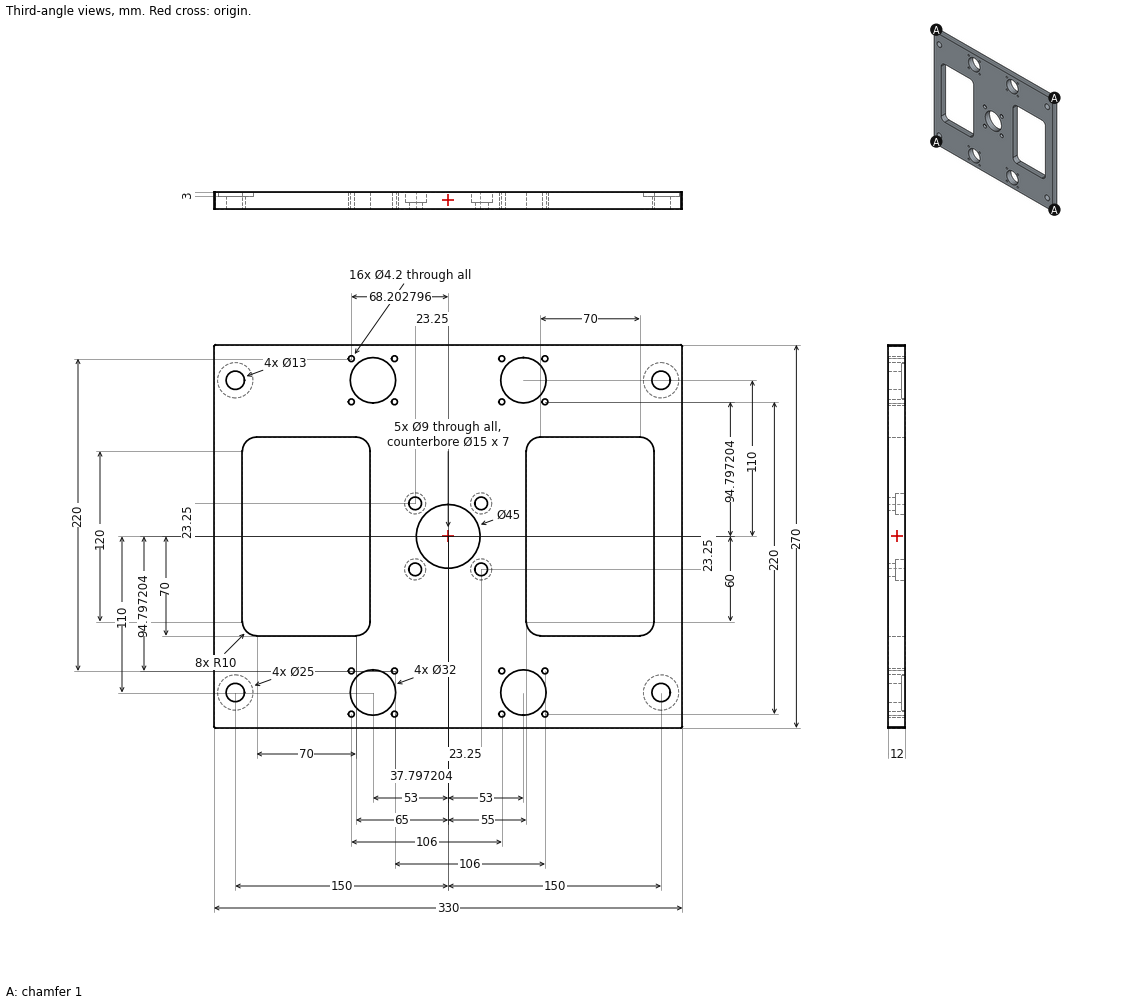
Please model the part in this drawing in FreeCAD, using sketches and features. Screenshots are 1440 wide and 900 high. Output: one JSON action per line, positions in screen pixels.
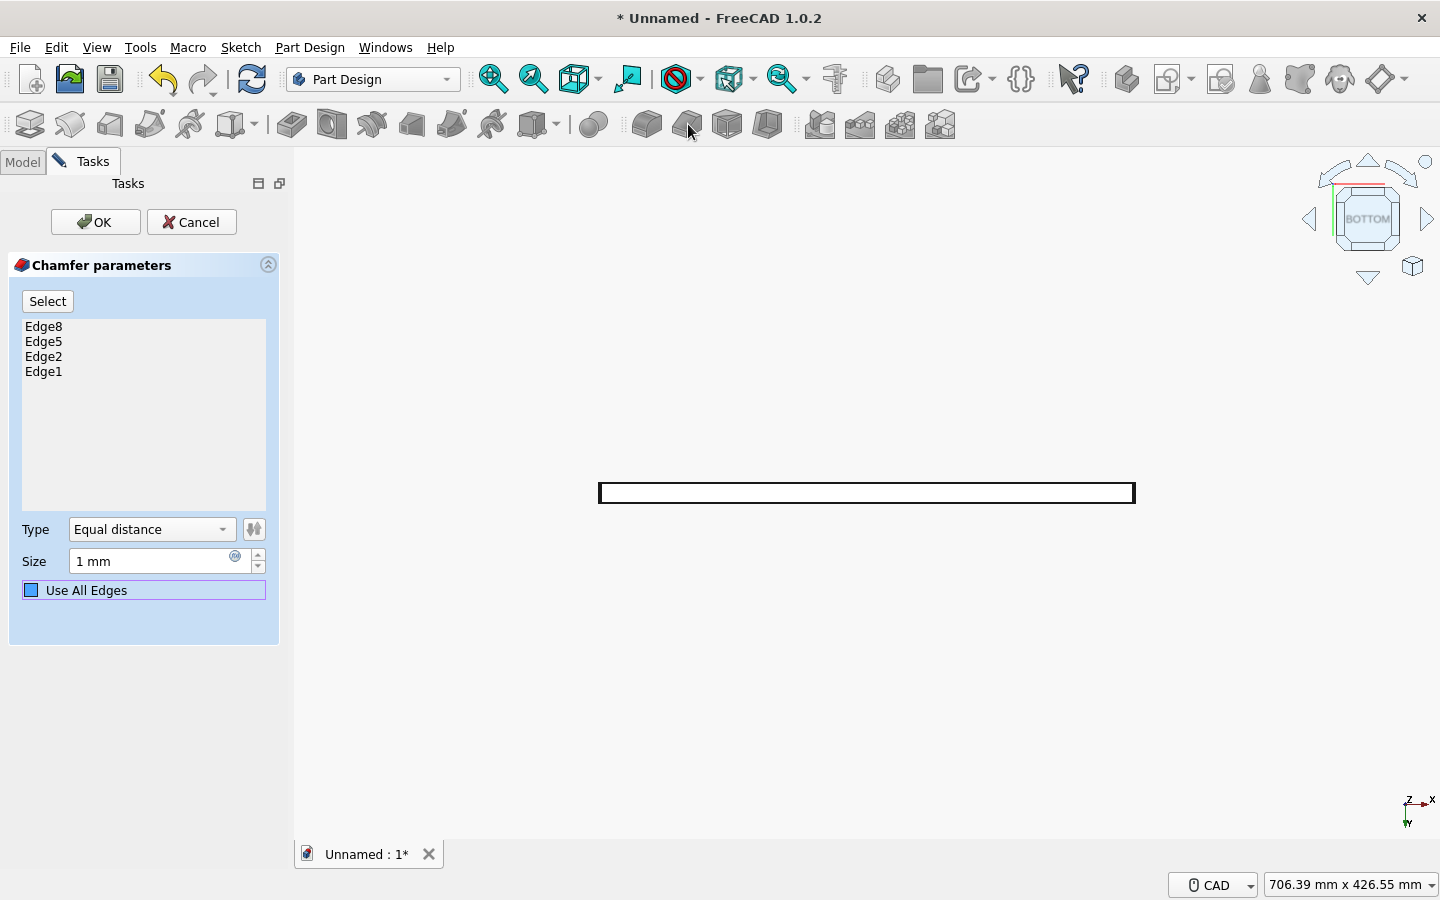
{"action": "left_click", "coordinate": [96, 222]}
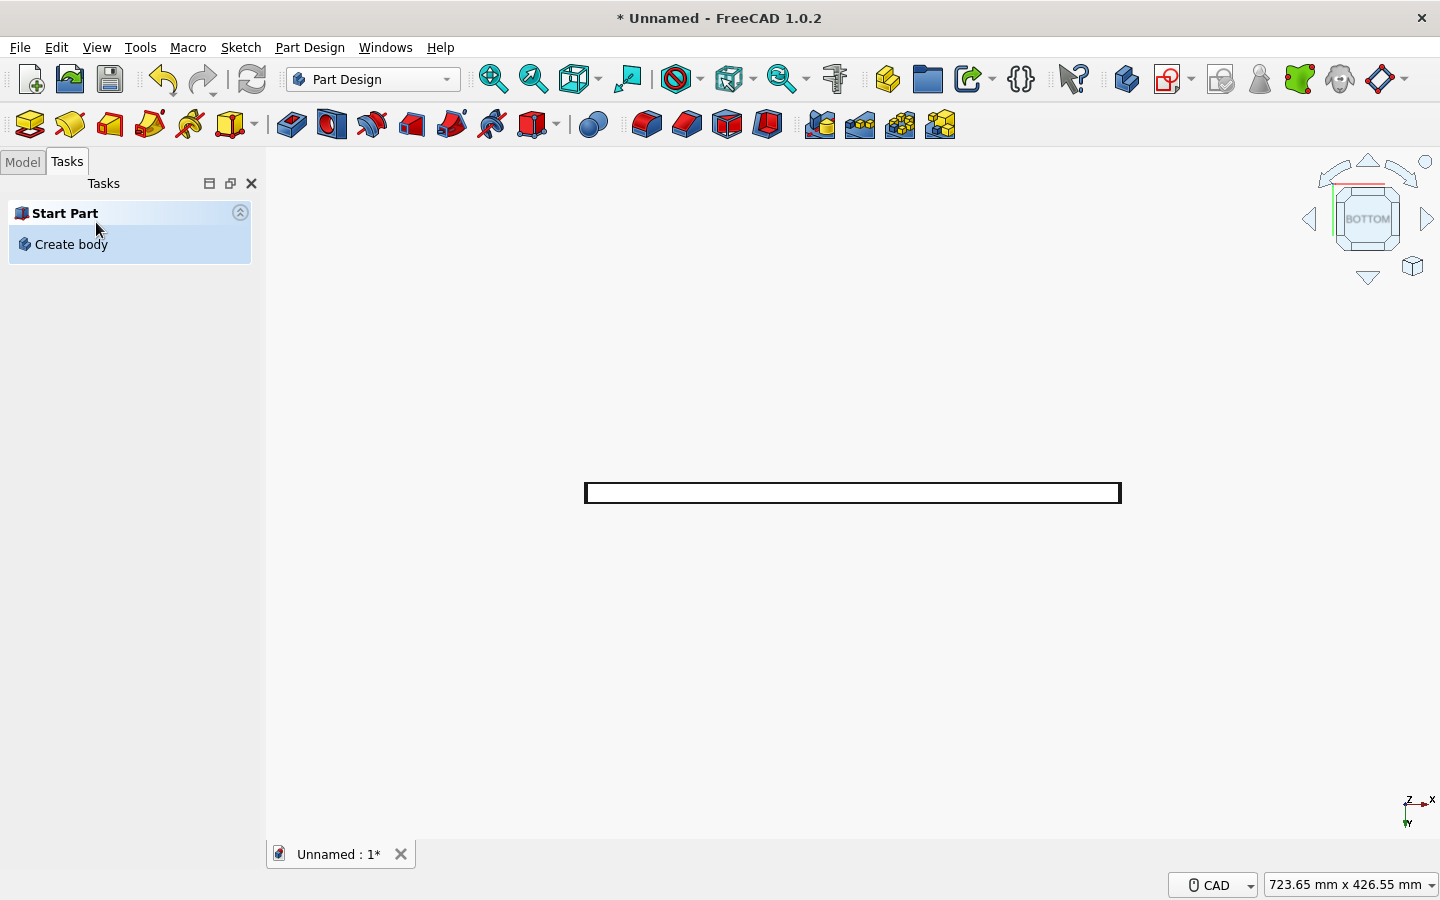
{"action": "key", "text": "4"}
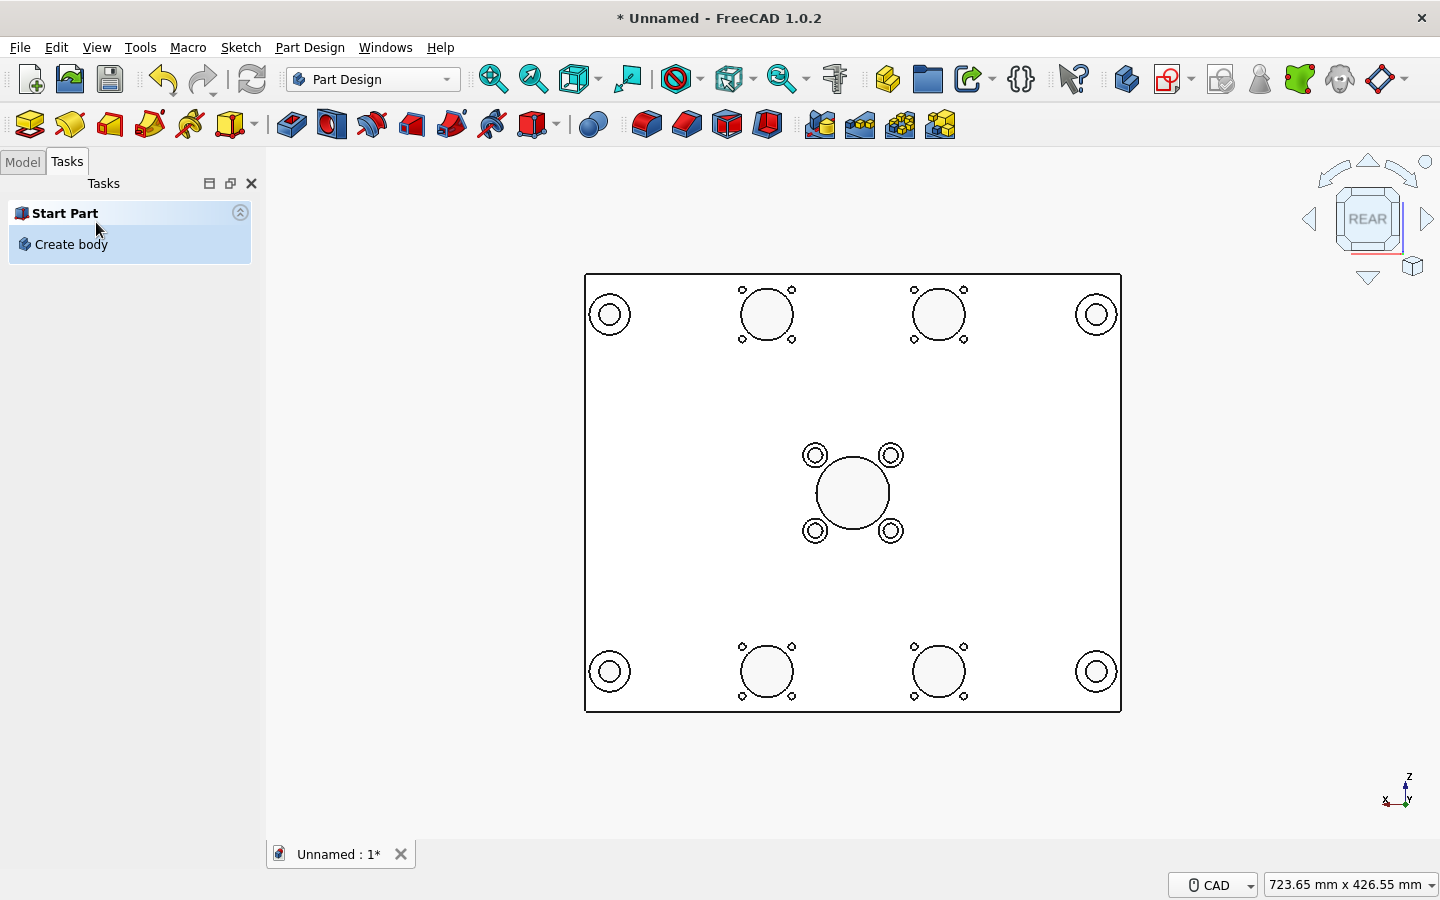
{"action": "left_click", "coordinate": [1006, 492]}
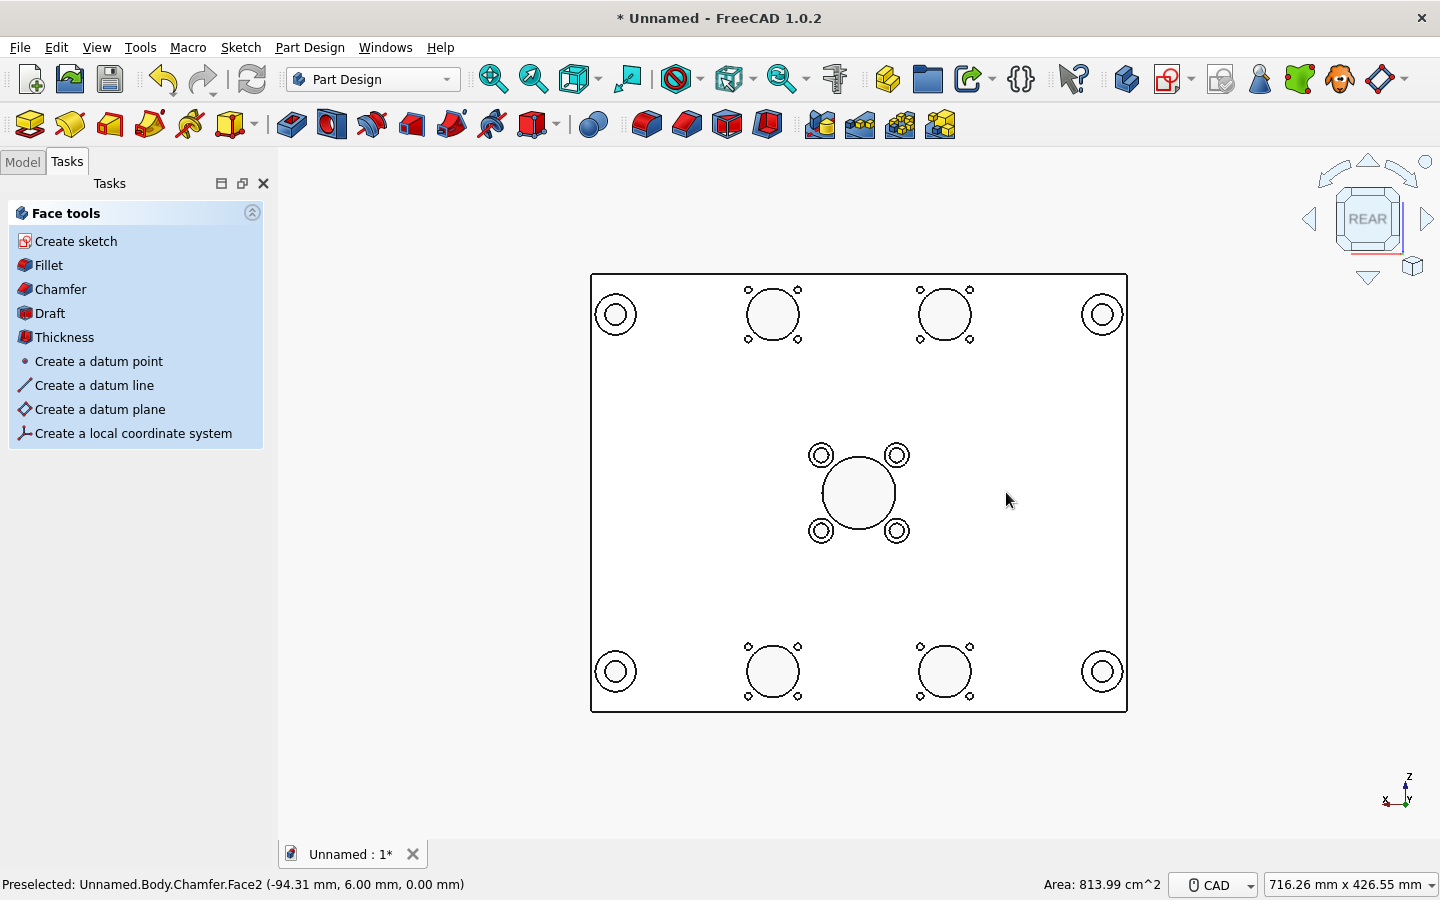
{"action": "left_click", "coordinate": [1168, 80]}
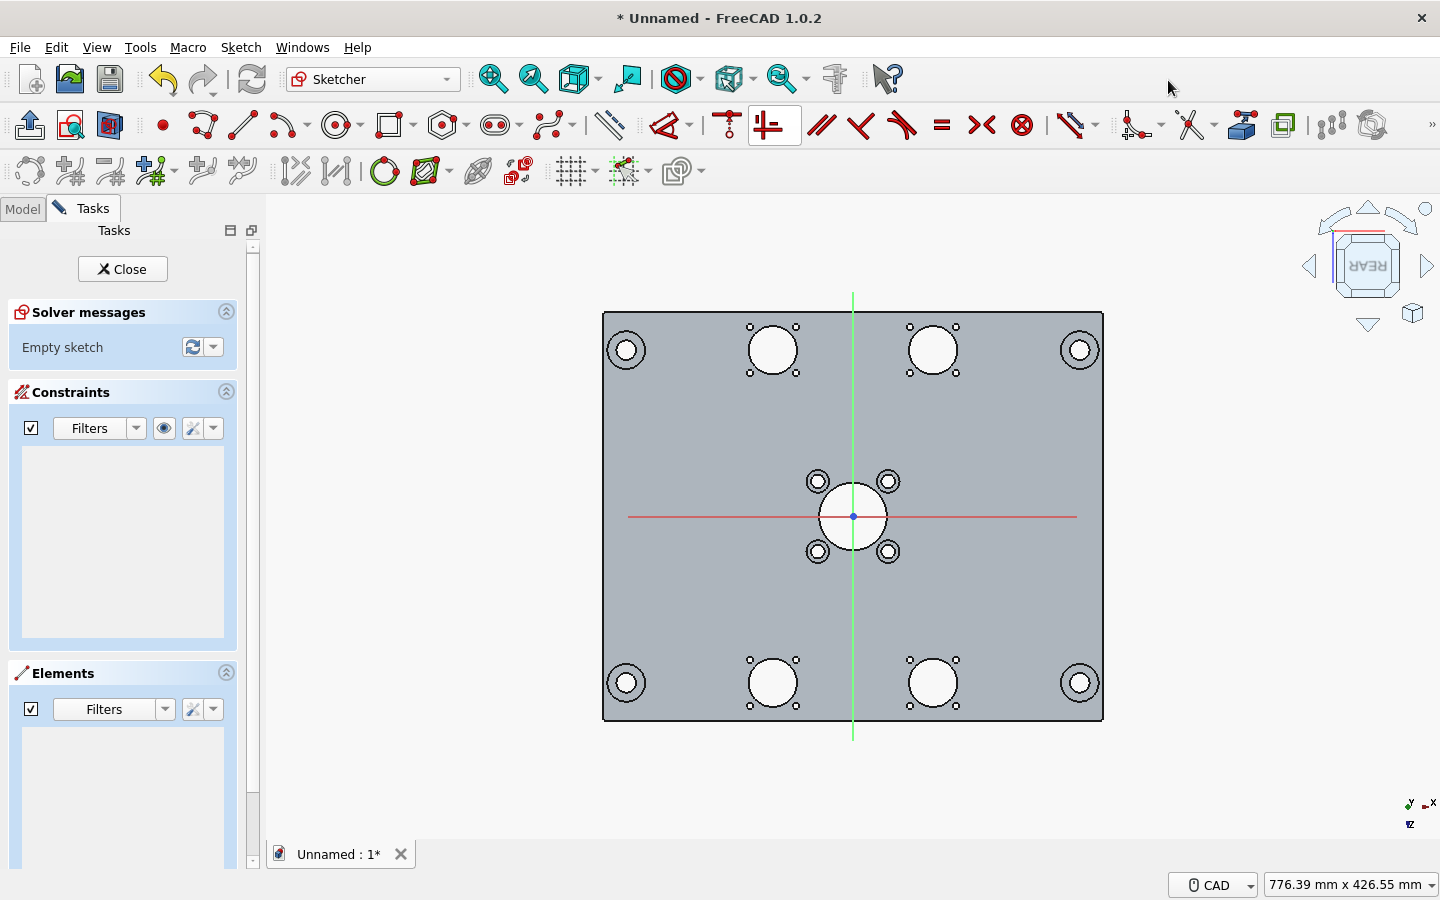
{"action": "scroll", "coordinate": [992, 517], "scroll_direction": "up", "scroll_amount": 2}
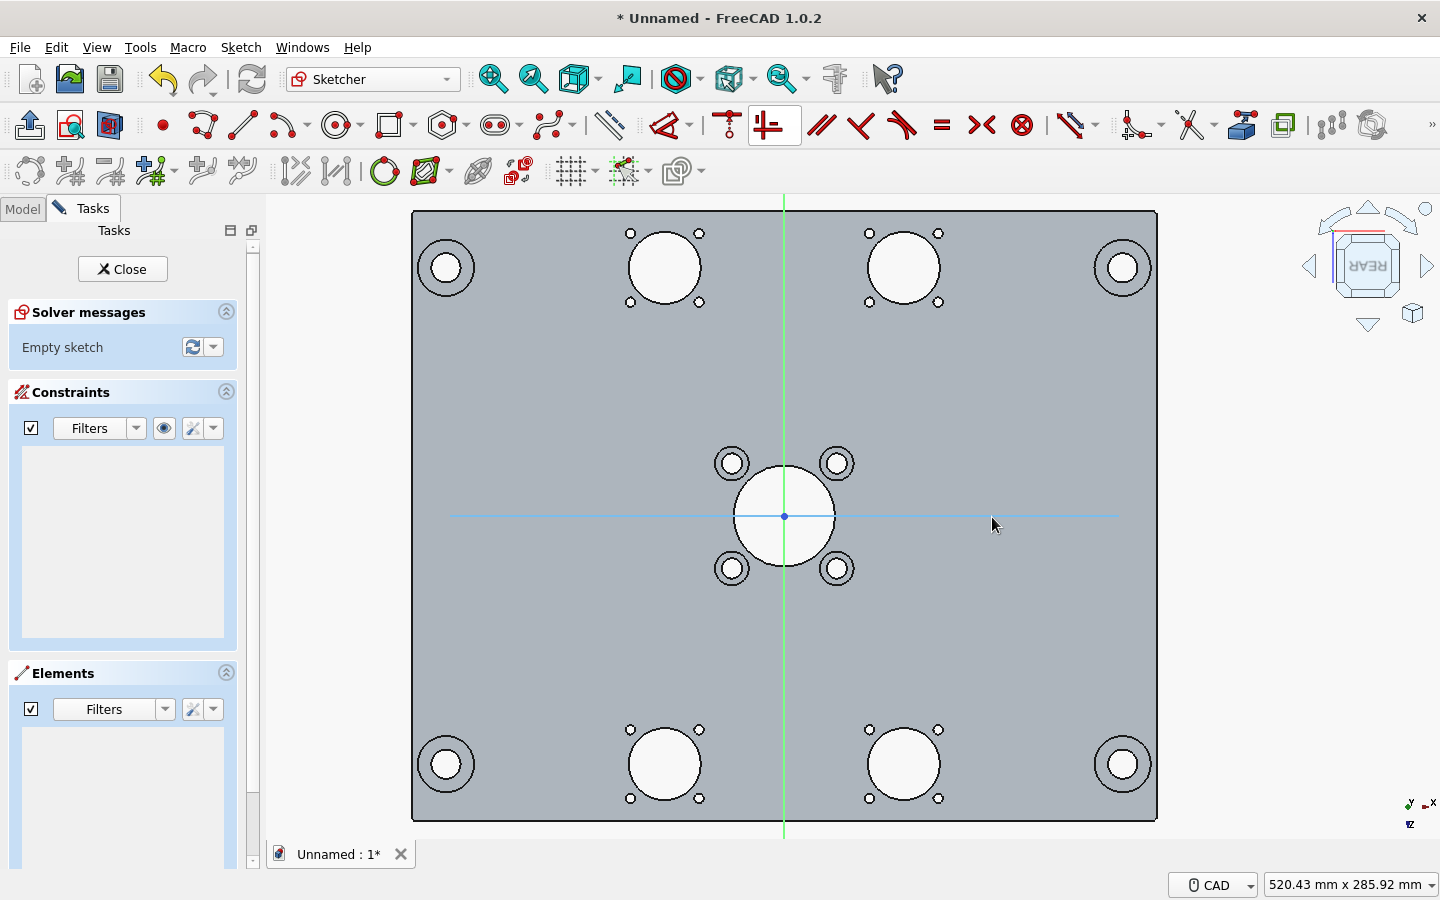
{"action": "left_click", "coordinate": [244, 126]}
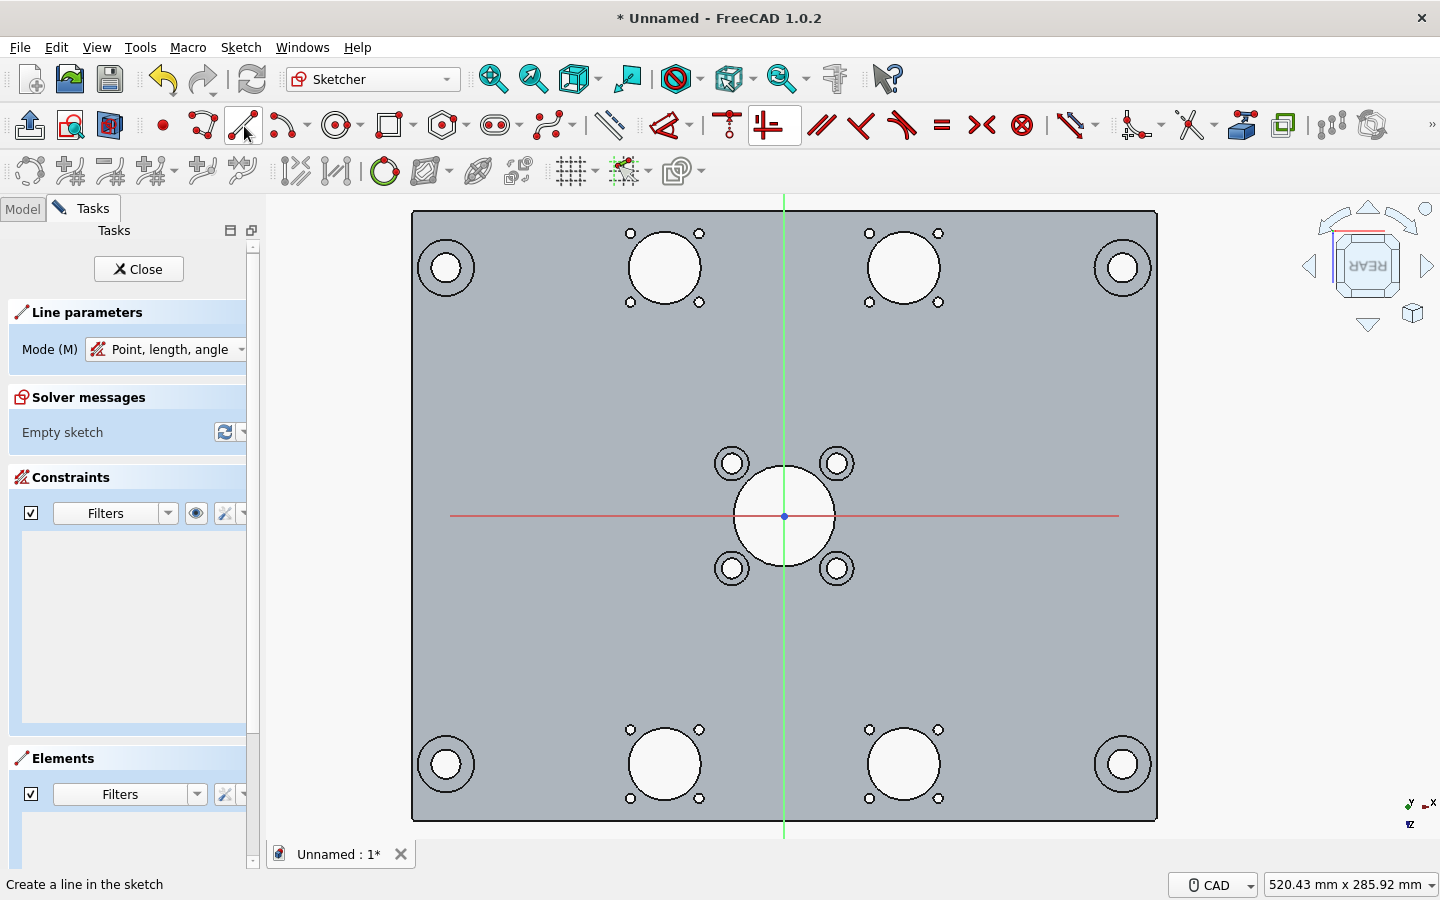
{"action": "left_click", "coordinate": [638, 358]}
{"action": "left_click", "coordinate": [480, 358]}